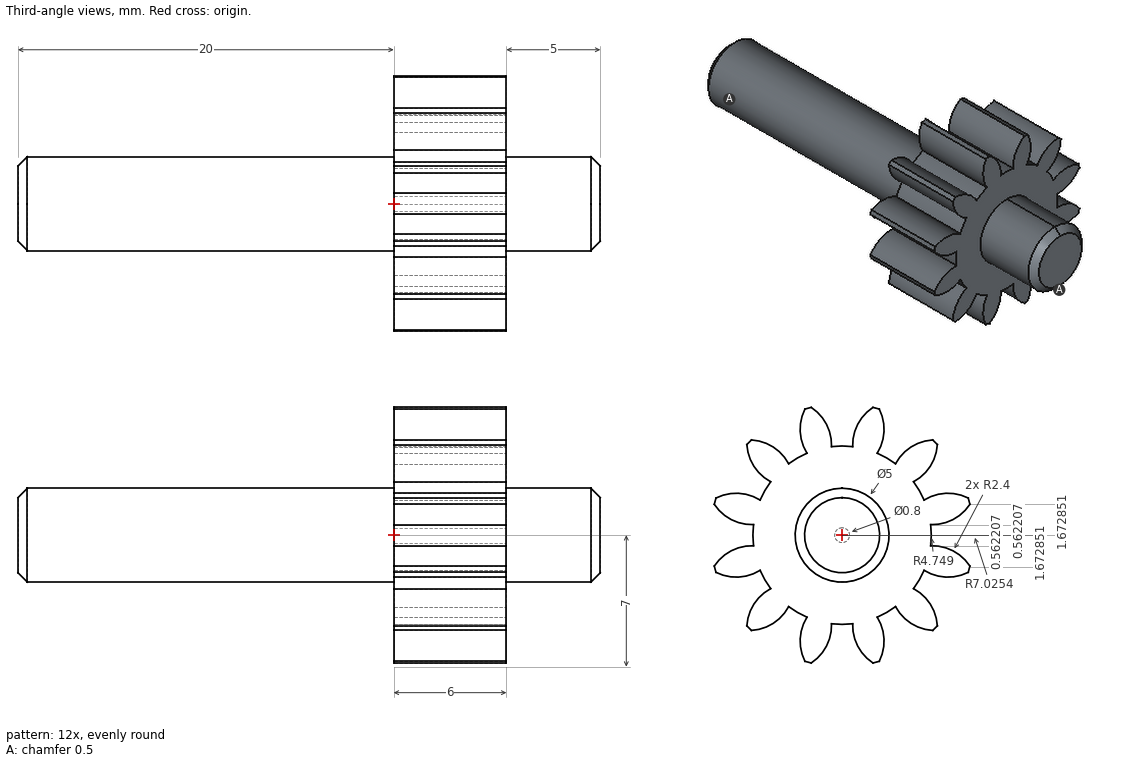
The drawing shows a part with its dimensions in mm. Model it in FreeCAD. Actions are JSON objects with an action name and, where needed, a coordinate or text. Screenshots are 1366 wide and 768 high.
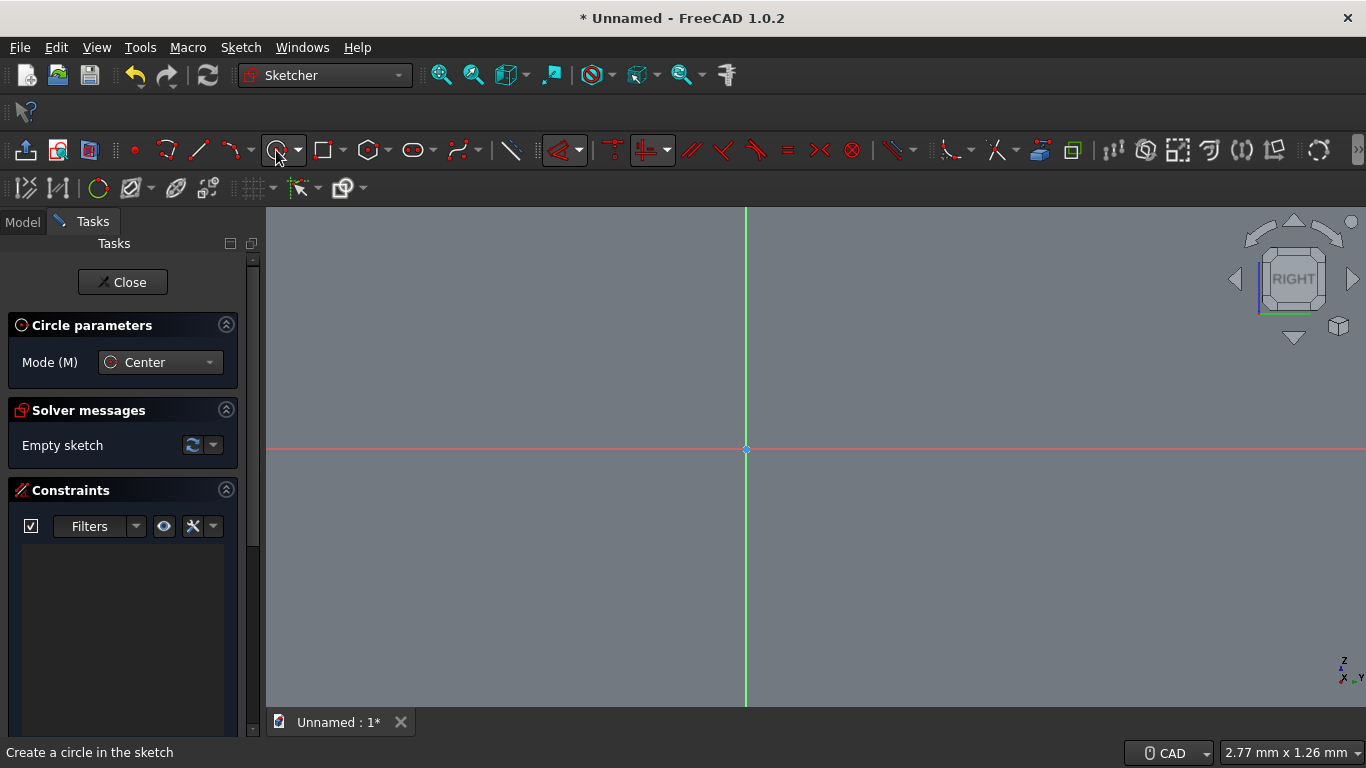
{"action": "left_click", "coordinate": [746, 449]}
{"action": "left_click", "coordinate": [859, 337]}
{"action": "key", "text": "Escape"}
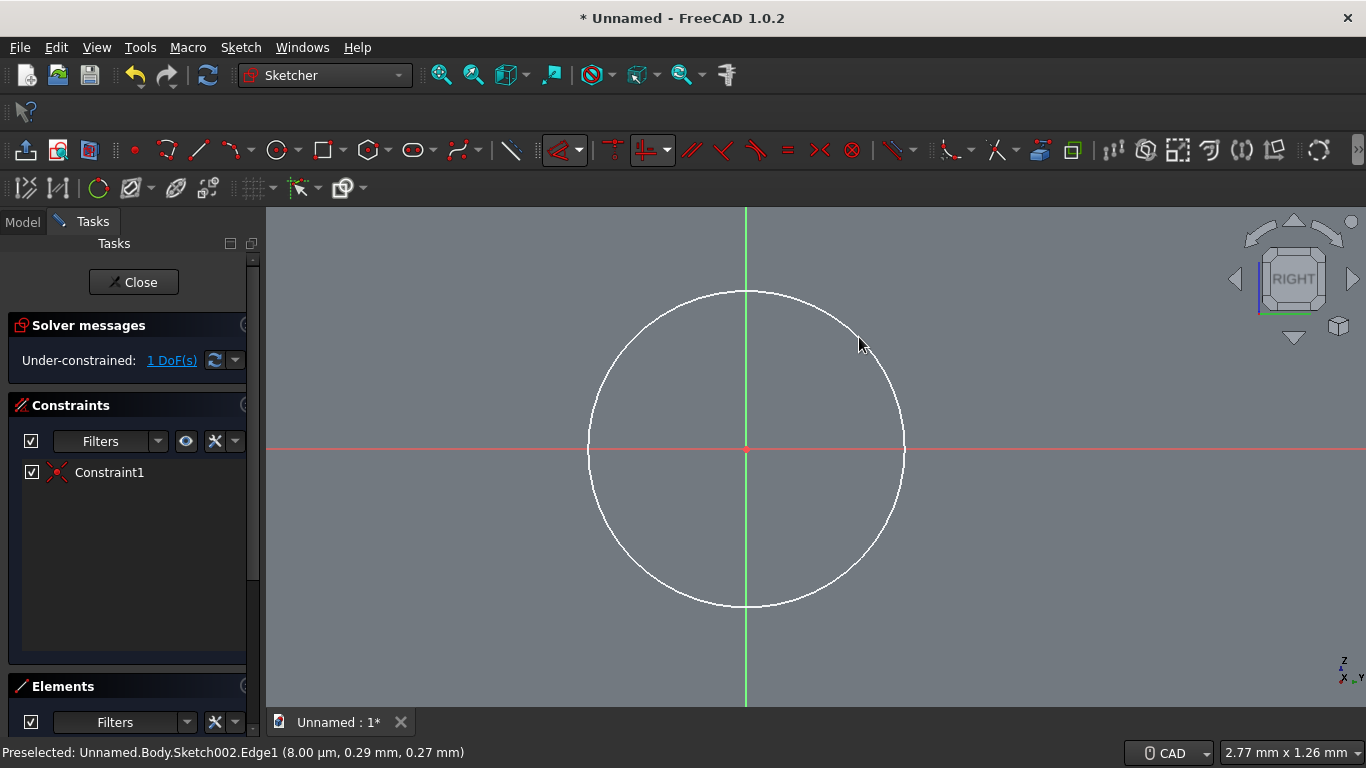
{"action": "left_click", "coordinate": [858, 337]}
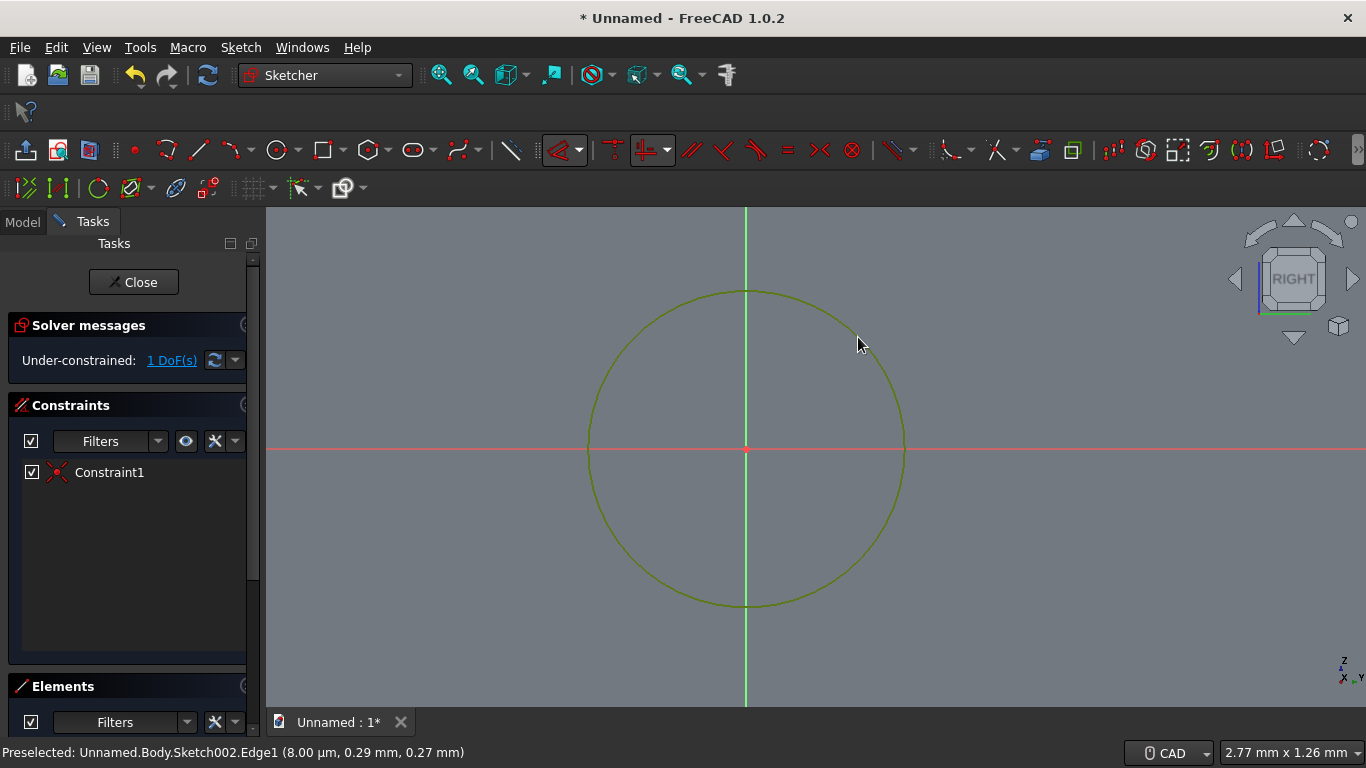
{"action": "left_click", "coordinate": [582, 150]}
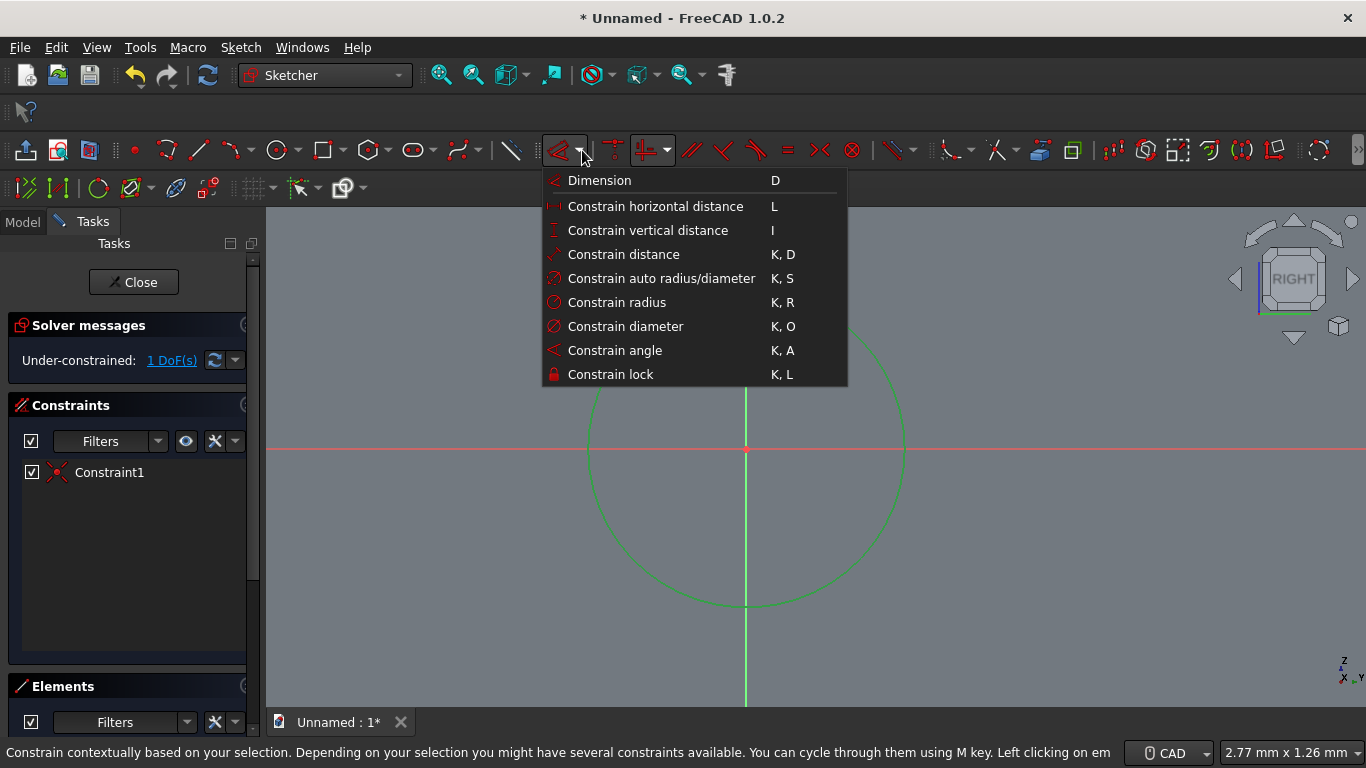
{"action": "left_click", "coordinate": [695, 326]}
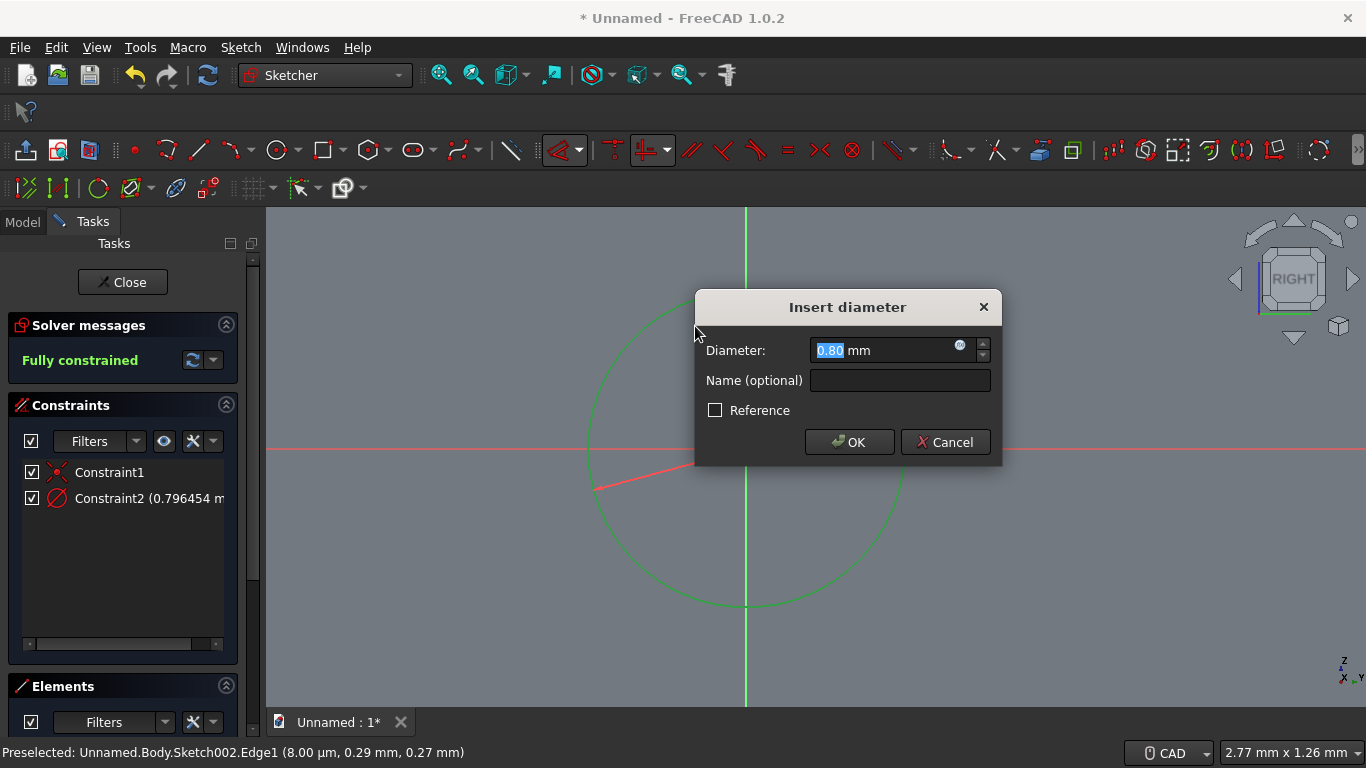
{"action": "type", "text": "0.8"}
{"action": "key", "text": "Return"}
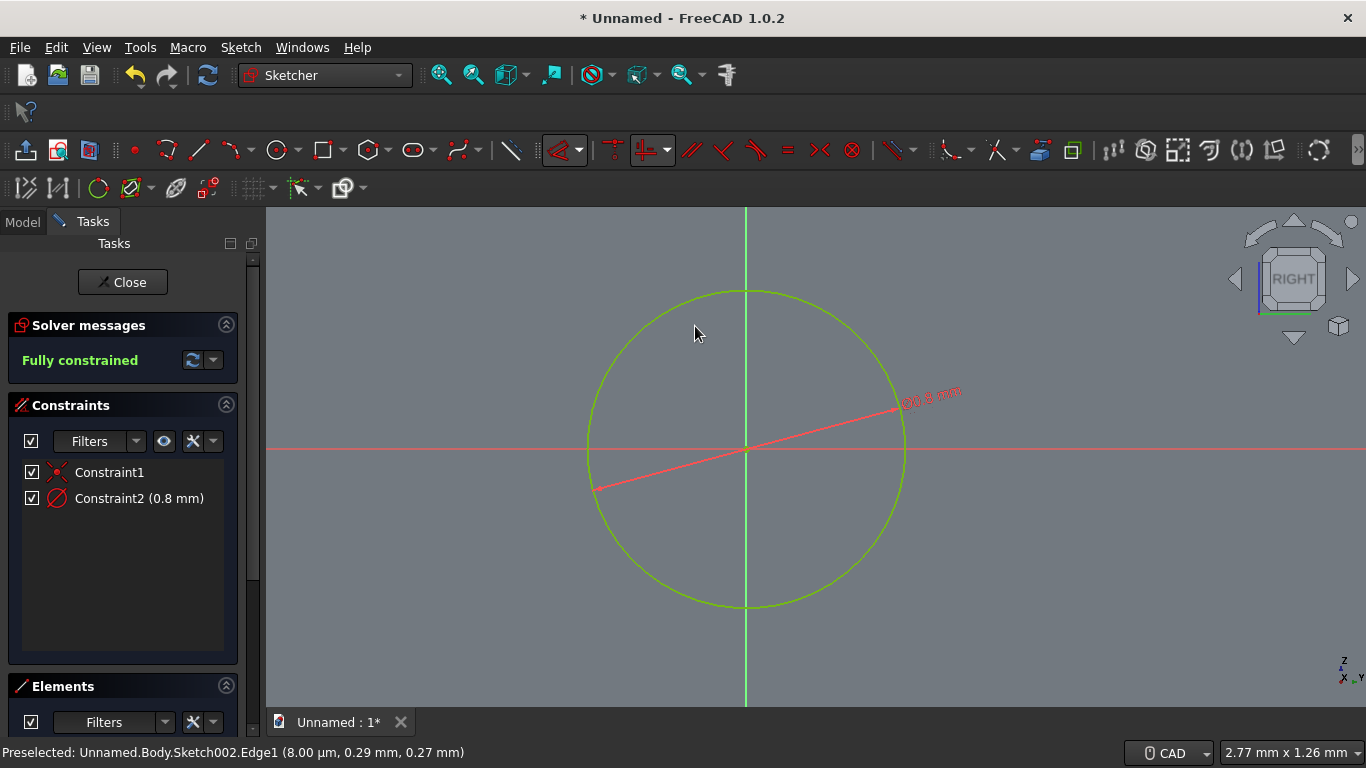
{"action": "left_click", "coordinate": [123, 282]}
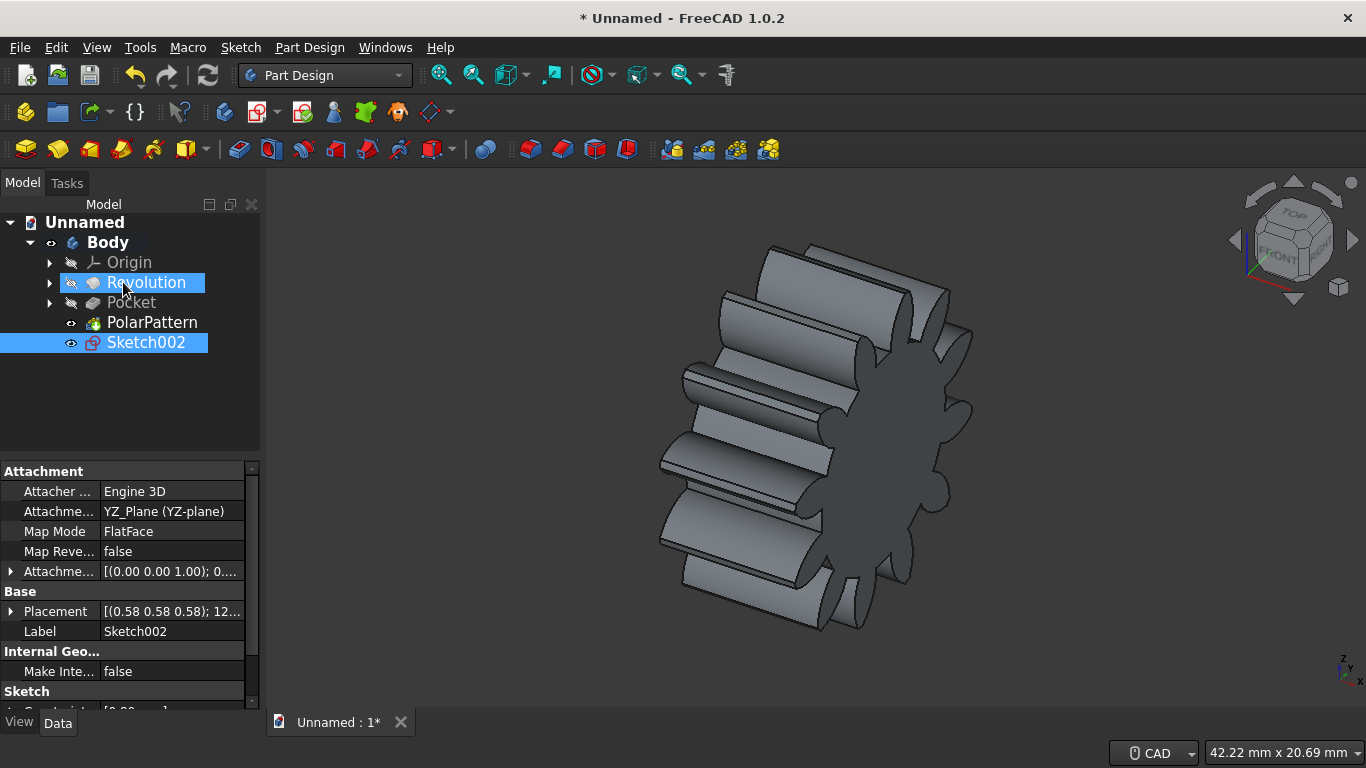
{"action": "left_click", "coordinate": [240, 150]}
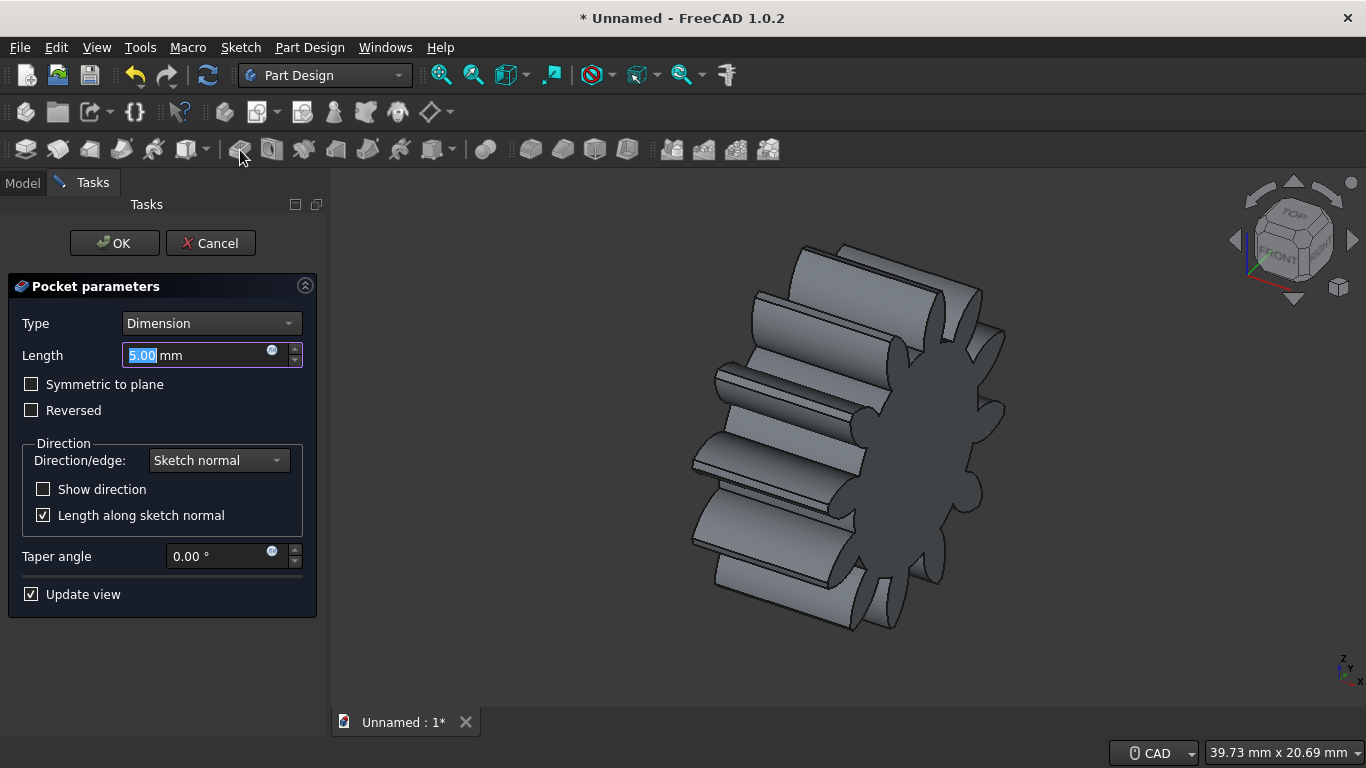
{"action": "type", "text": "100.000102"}
{"action": "key", "text": "Tab"}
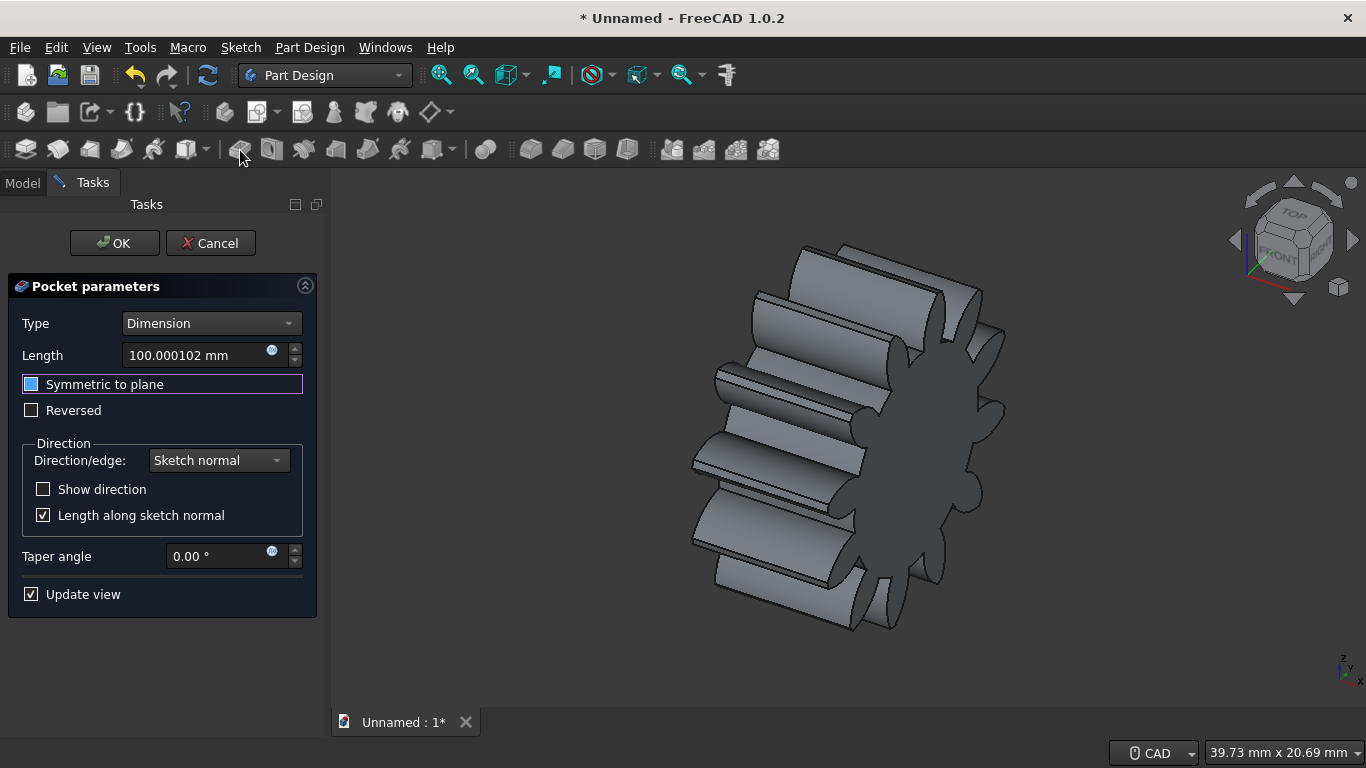
{"action": "left_click", "coordinate": [30, 384]}